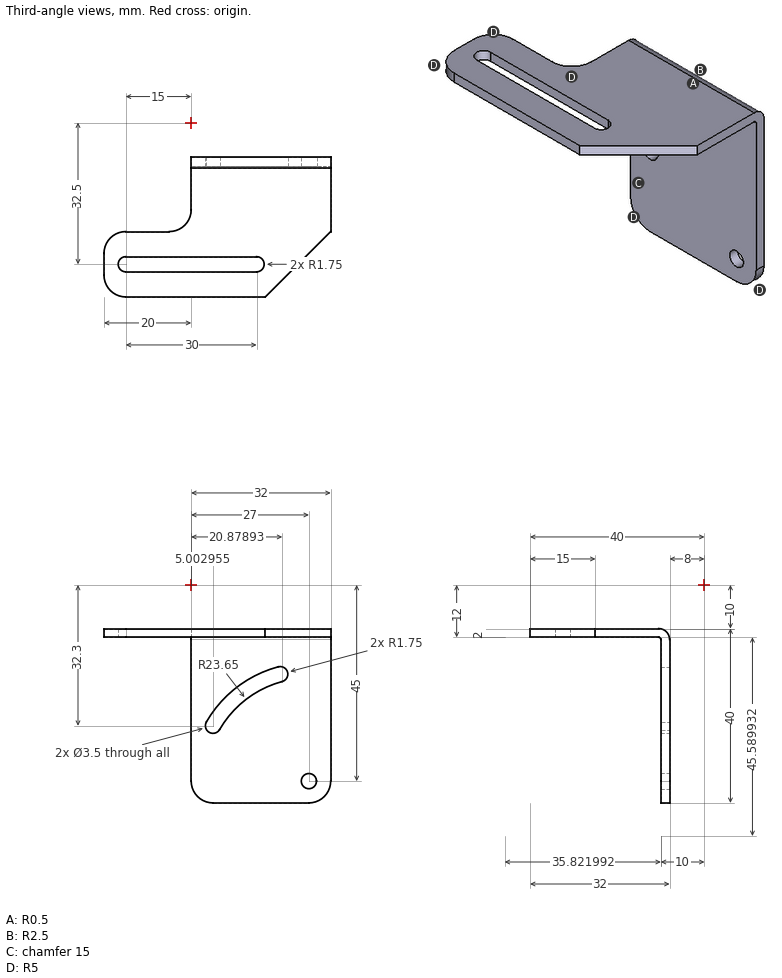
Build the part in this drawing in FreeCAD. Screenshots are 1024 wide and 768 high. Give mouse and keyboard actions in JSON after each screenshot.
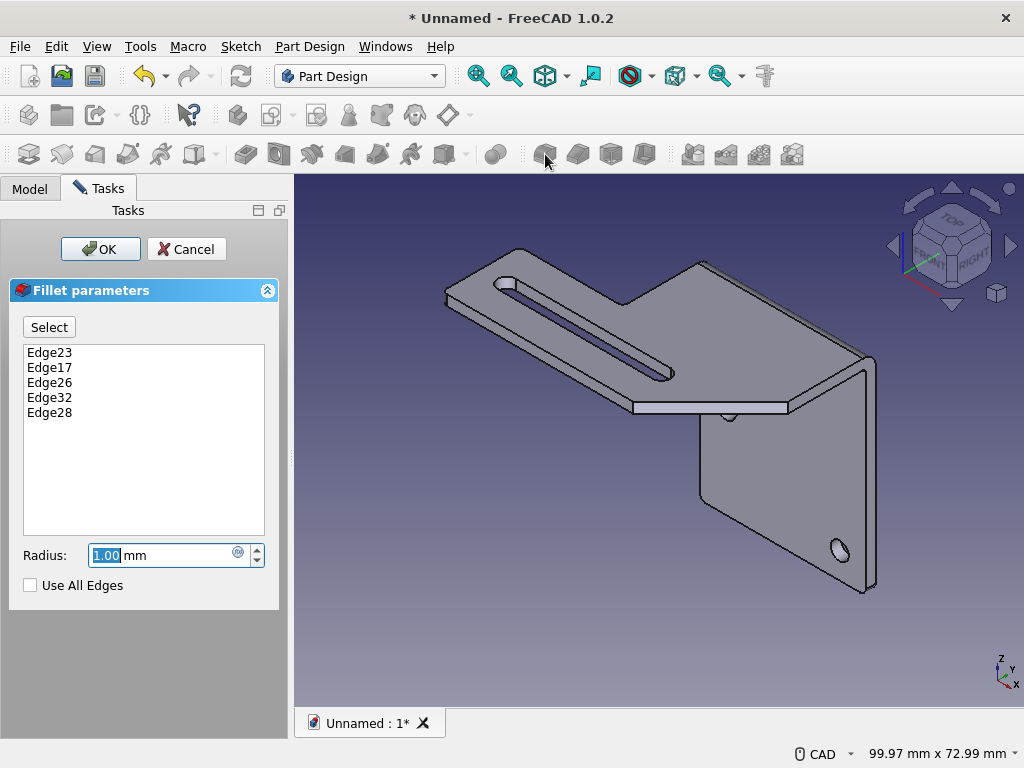
{"action": "type", "text": "5"}
{"action": "key", "text": "Tab"}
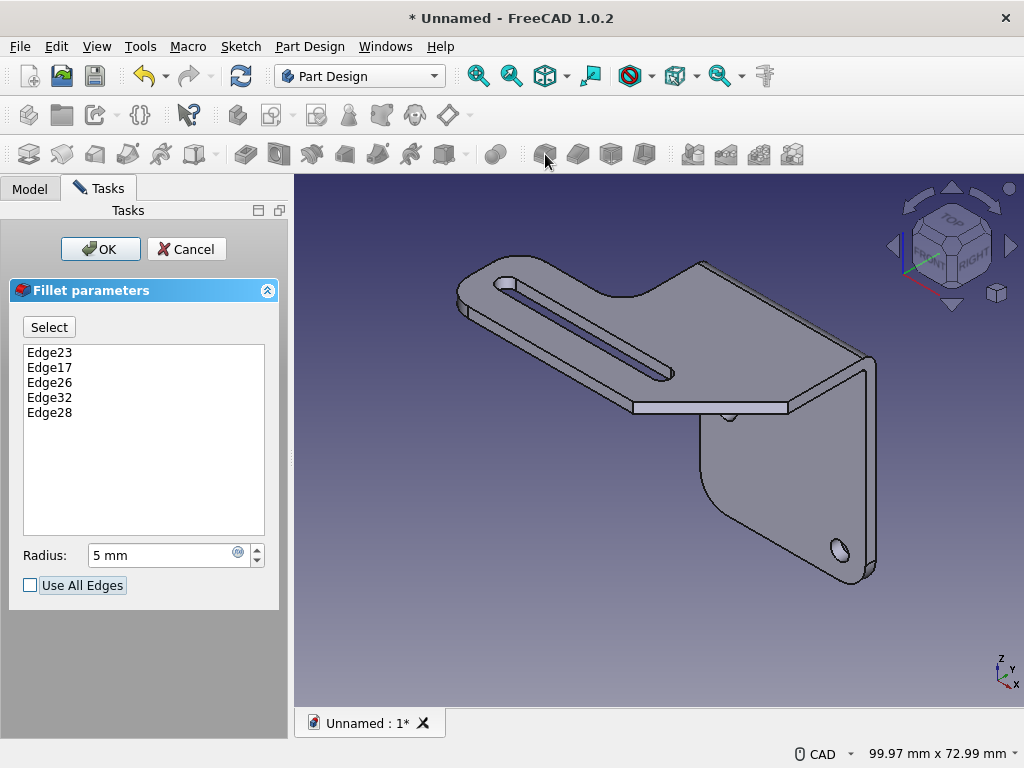
{"action": "left_click", "coordinate": [101, 249]}